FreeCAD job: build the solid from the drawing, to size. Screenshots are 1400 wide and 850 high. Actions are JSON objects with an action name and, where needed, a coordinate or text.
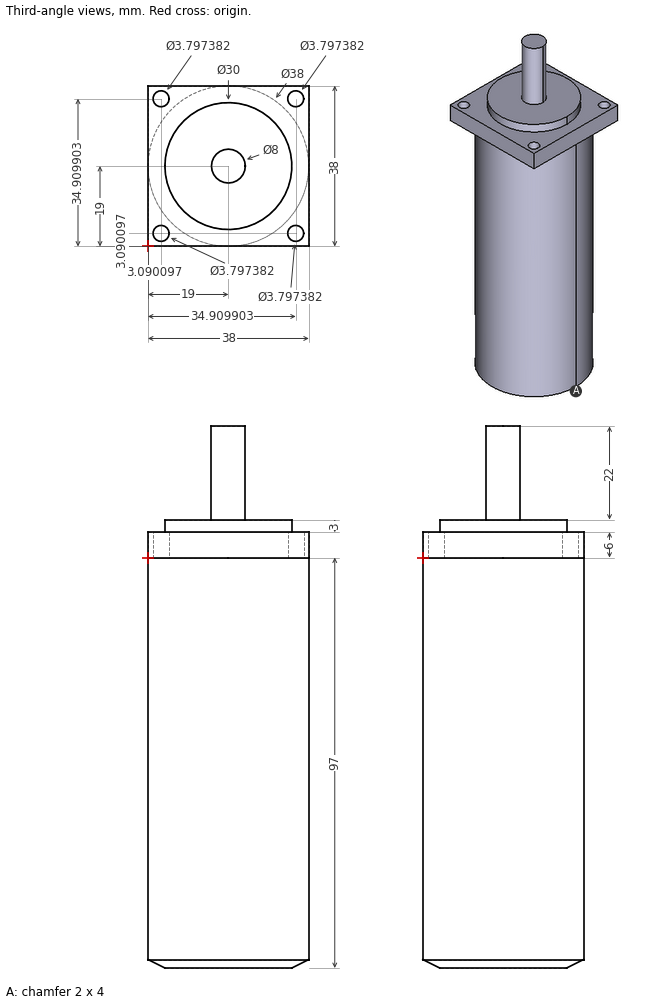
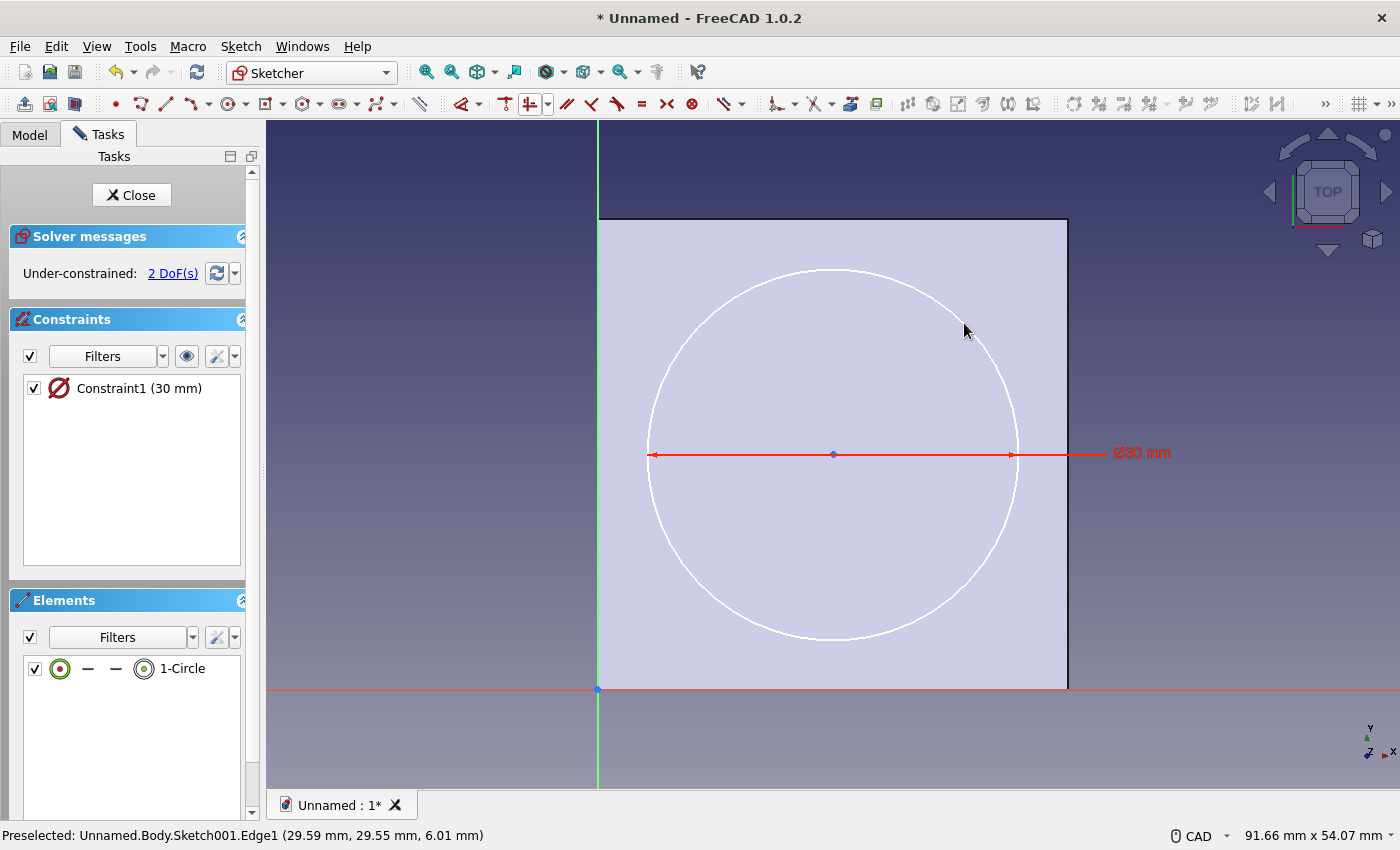
{"action": "key", "text": "d"}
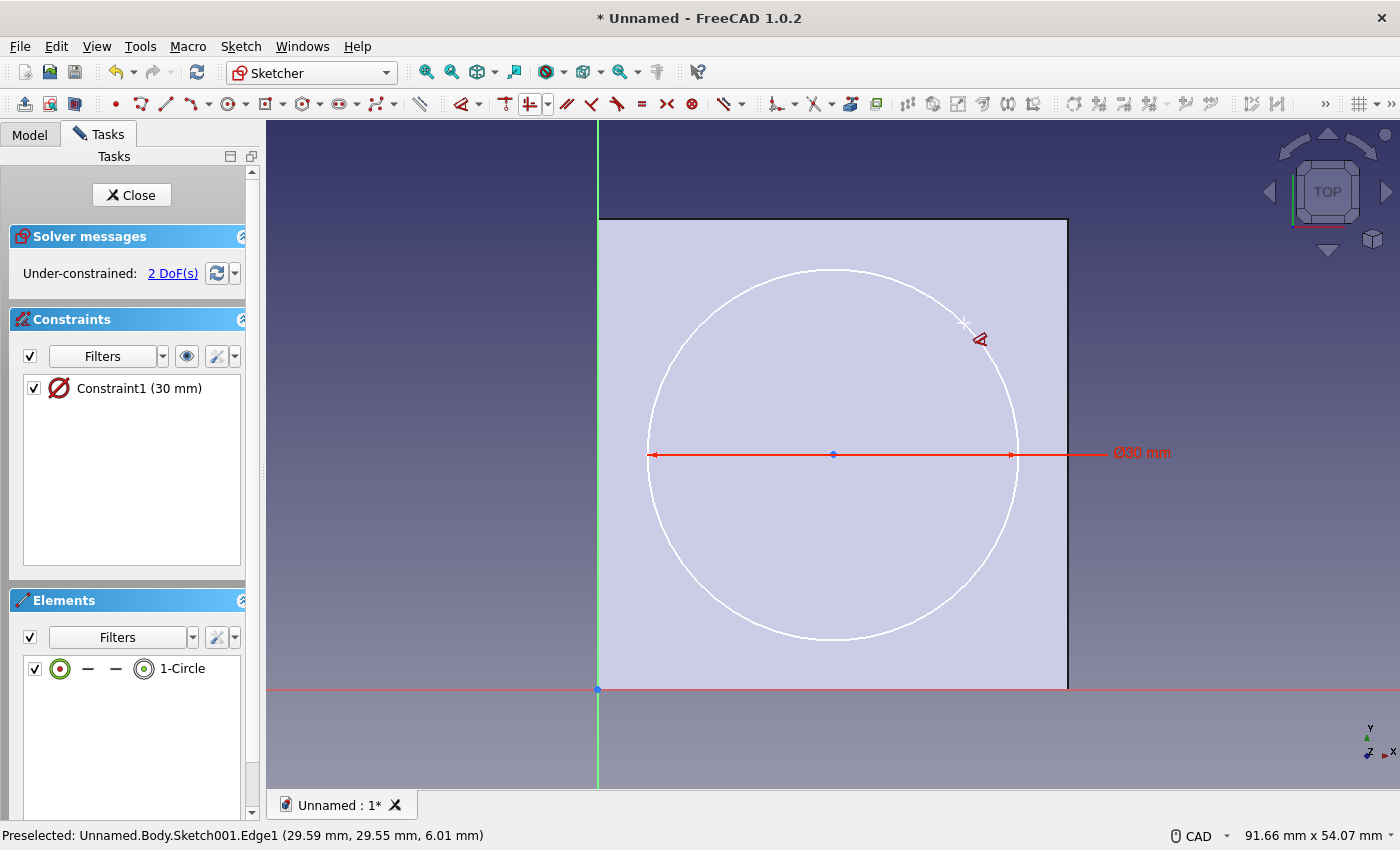
{"action": "left_click", "coordinate": [833, 455]}
{"action": "left_click", "coordinate": [715, 724]}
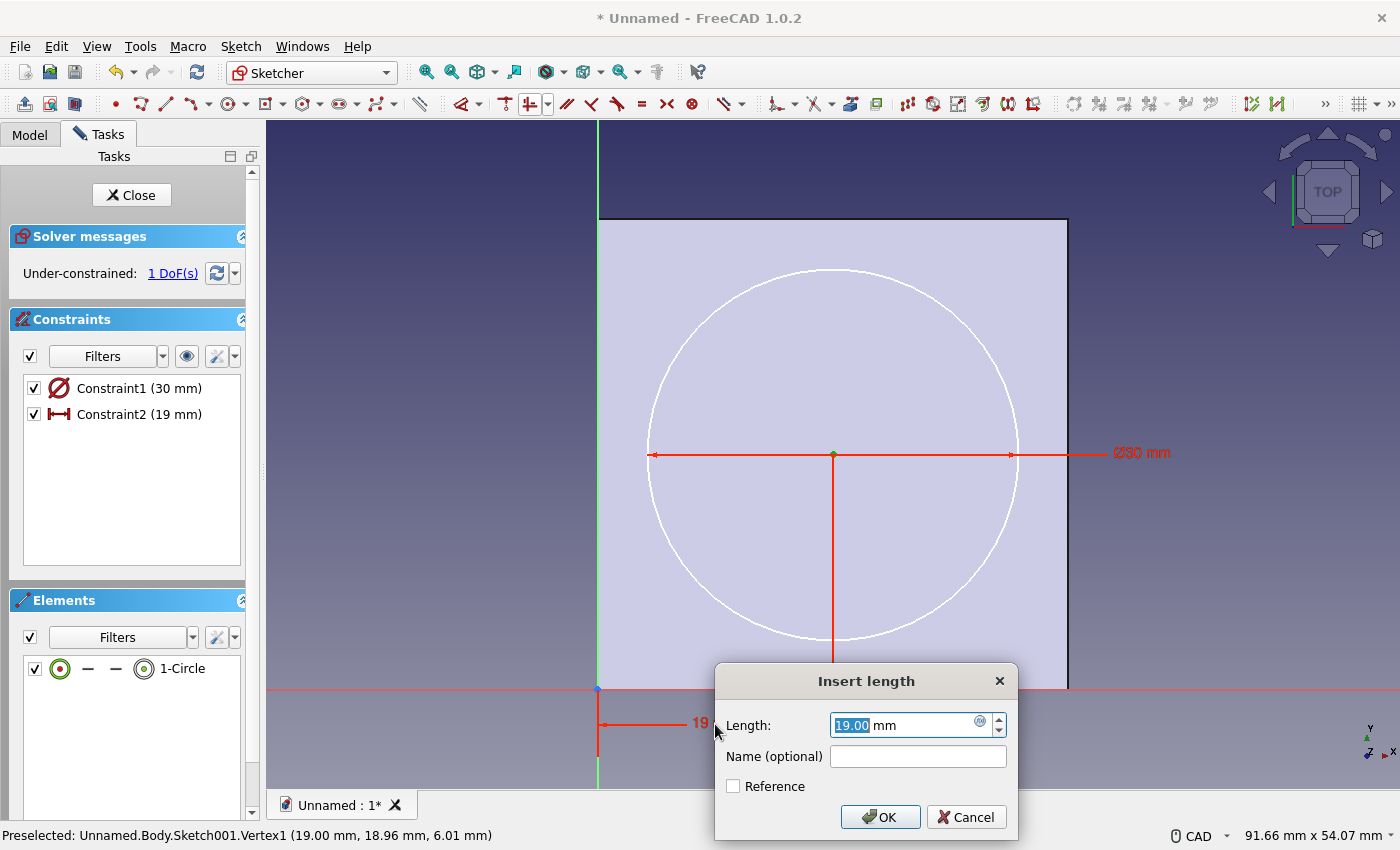
{"action": "type", "text": "19"}
{"action": "key", "text": "Return"}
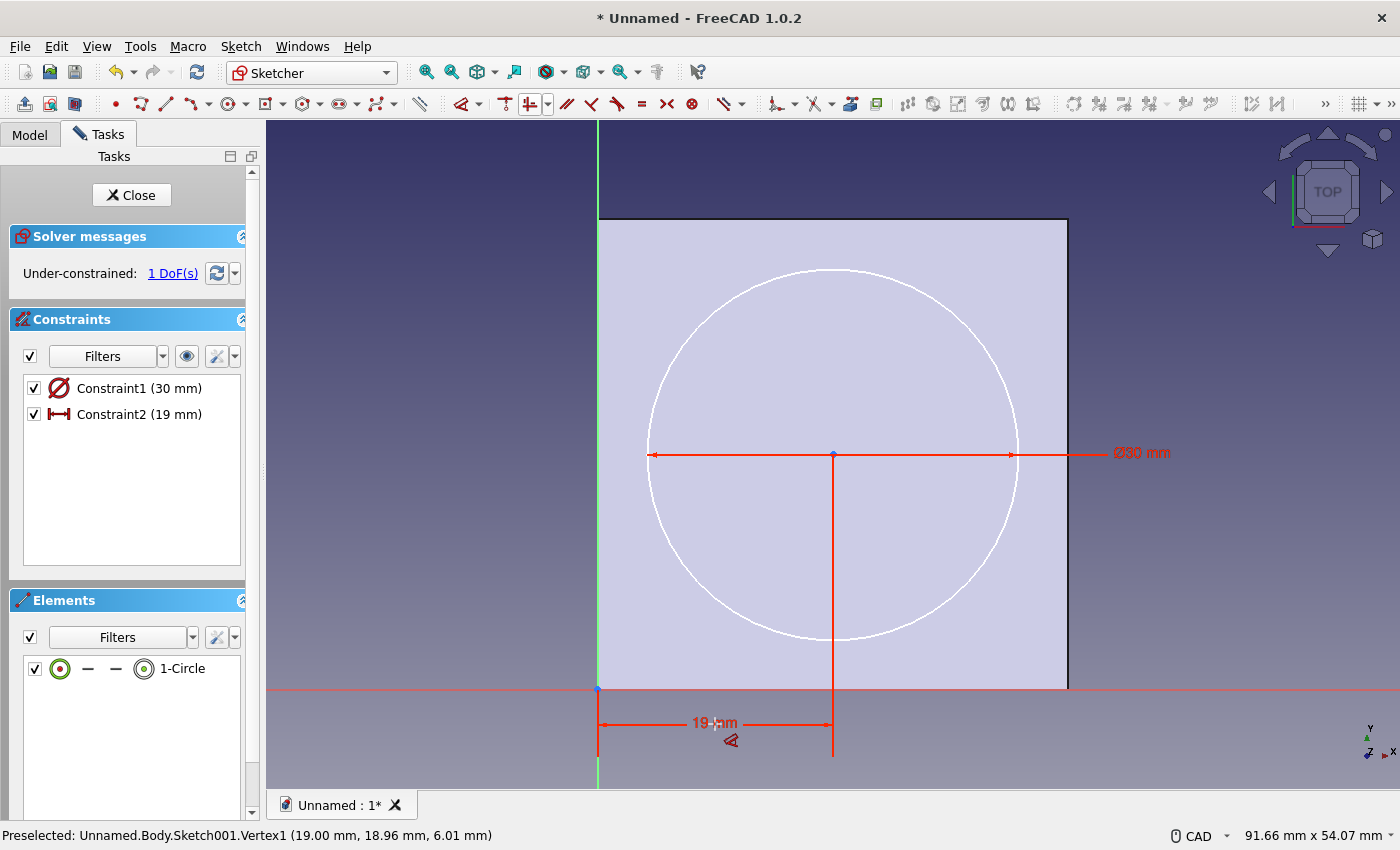
{"action": "left_click", "coordinate": [833, 455]}
{"action": "left_click", "coordinate": [564, 572]}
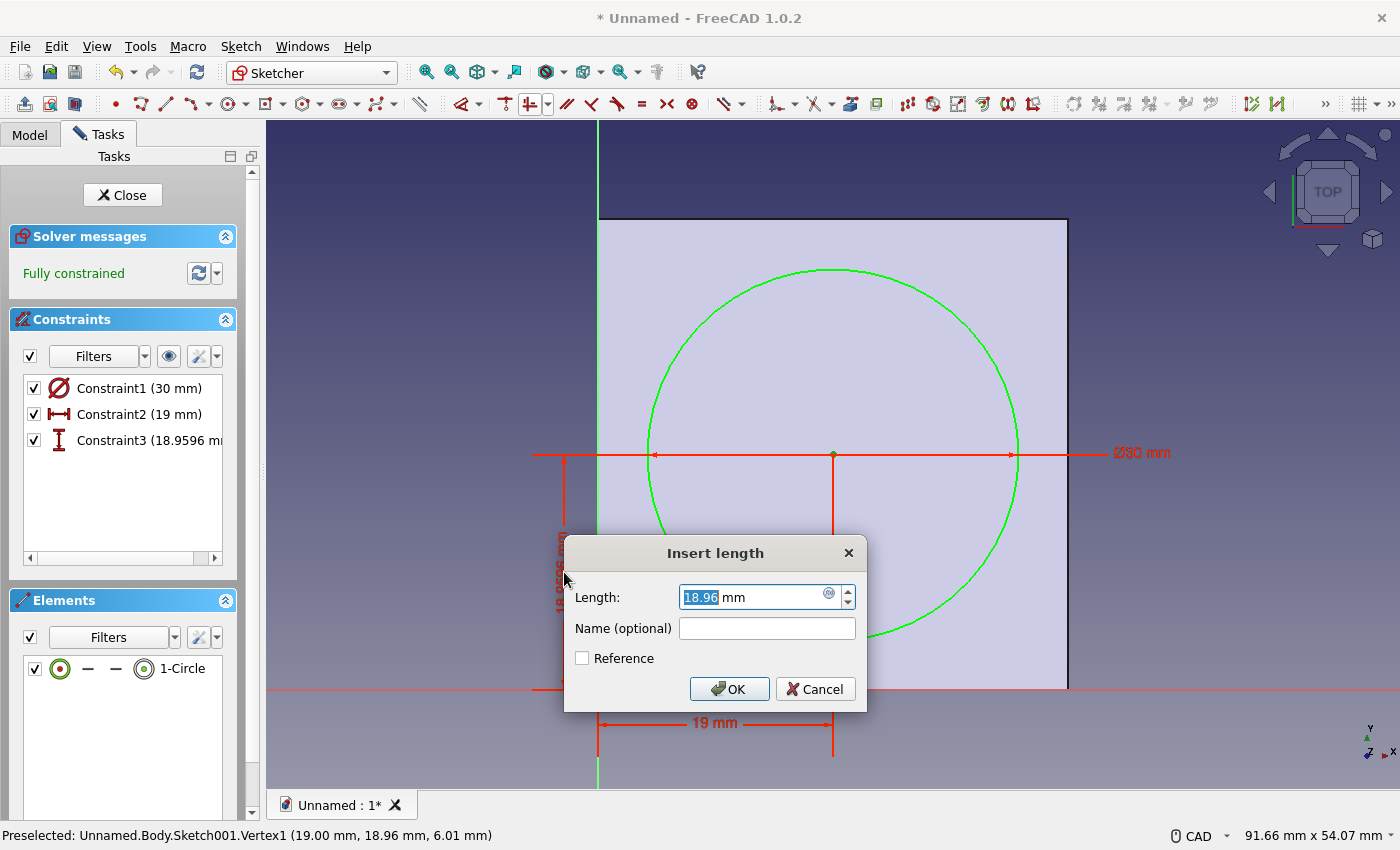
{"action": "type", "text": "19"}
{"action": "key", "text": "Return"}
{"action": "key", "text": "Escape"}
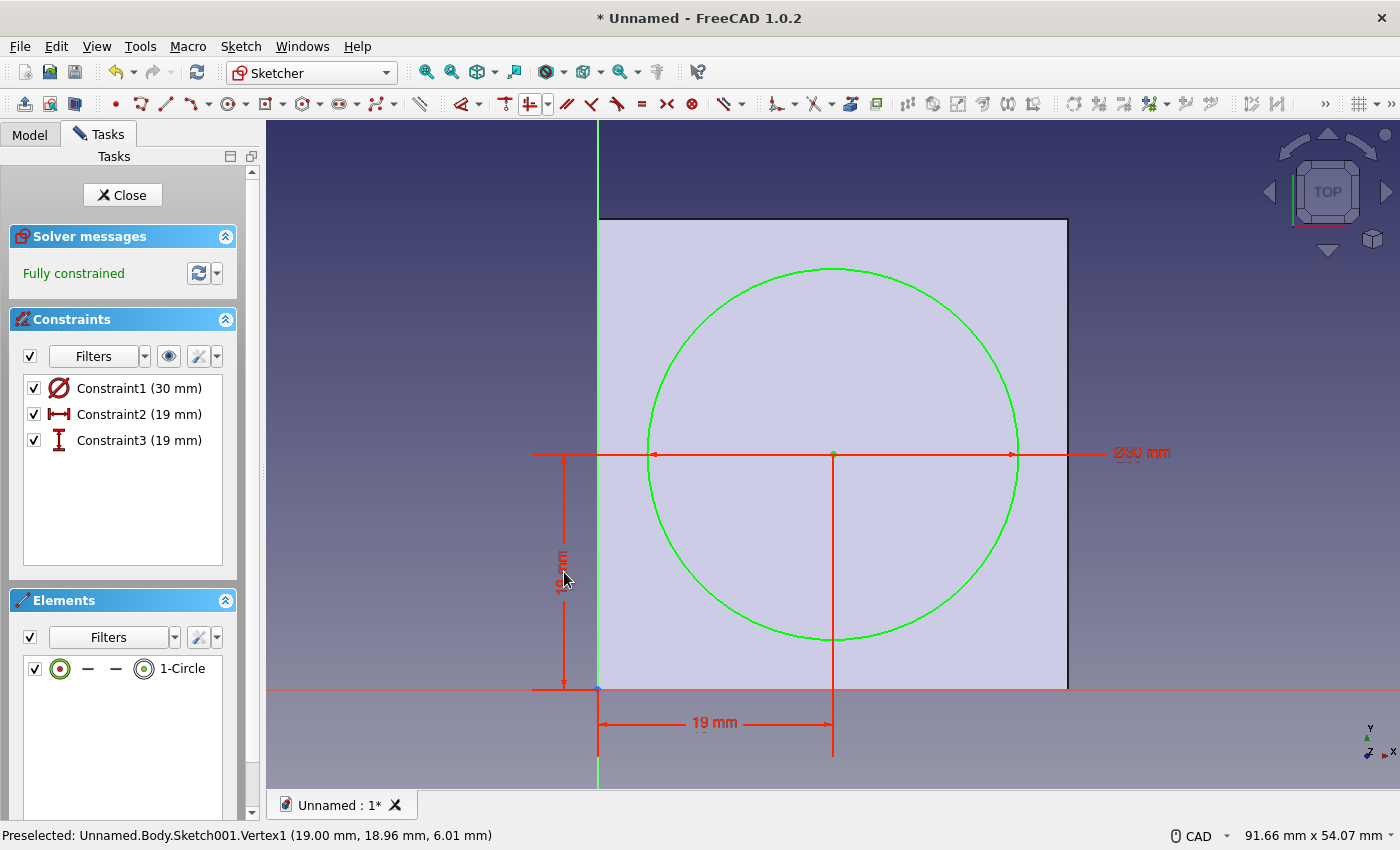
{"action": "left_click", "coordinate": [123, 195]}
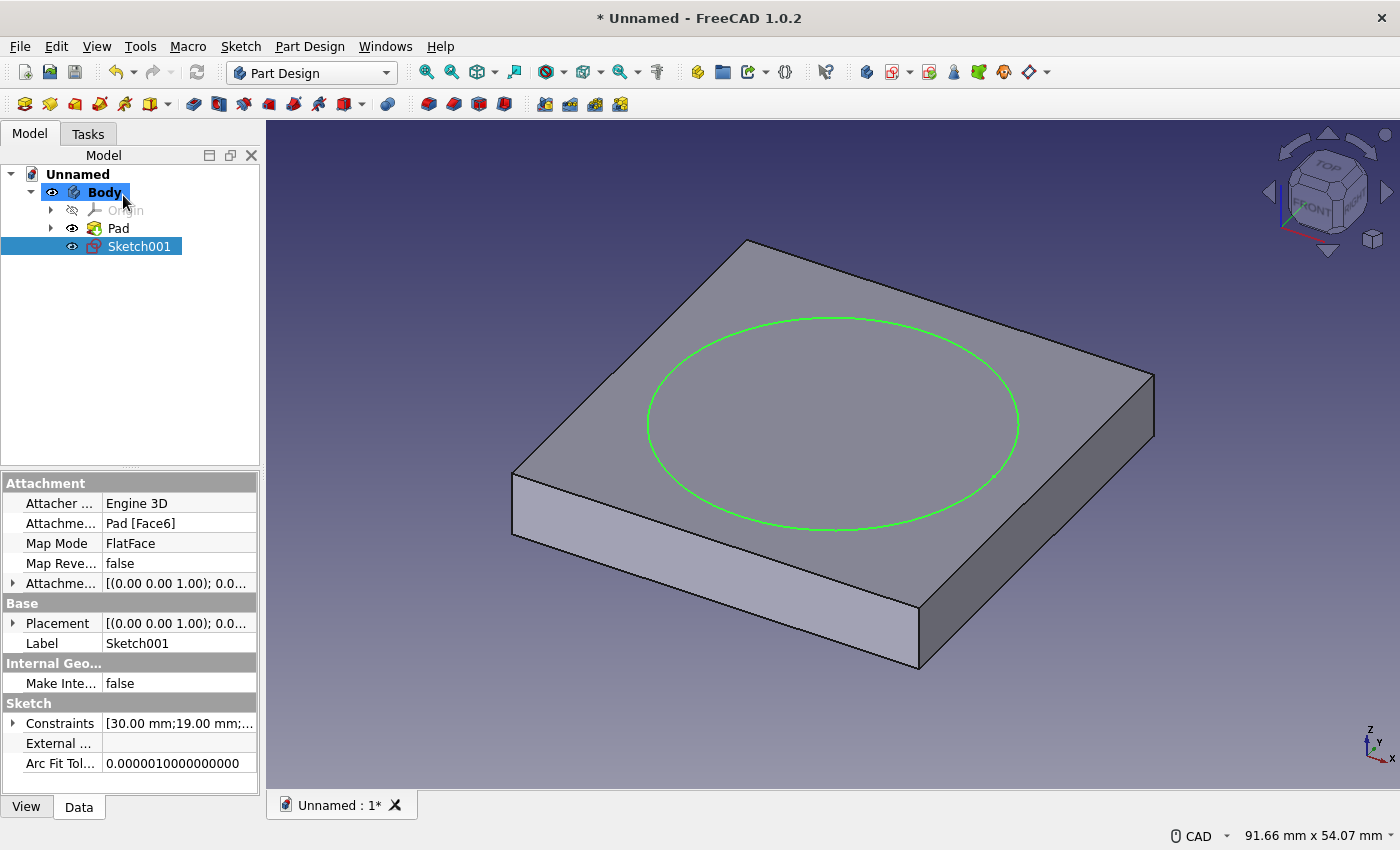
{"action": "left_click", "coordinate": [25, 104]}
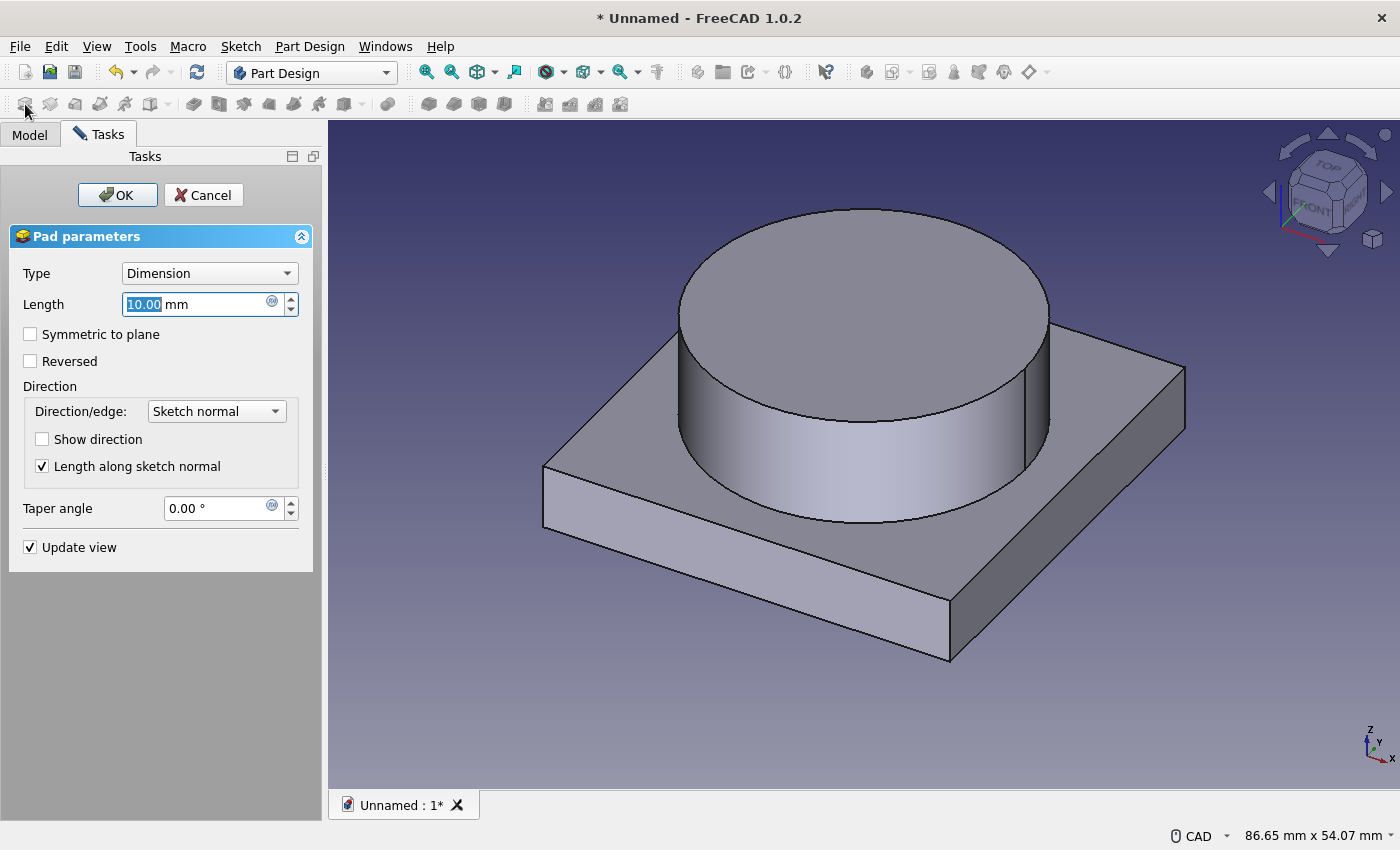
{"action": "type", "text": "3"}
{"action": "key", "text": "Tab"}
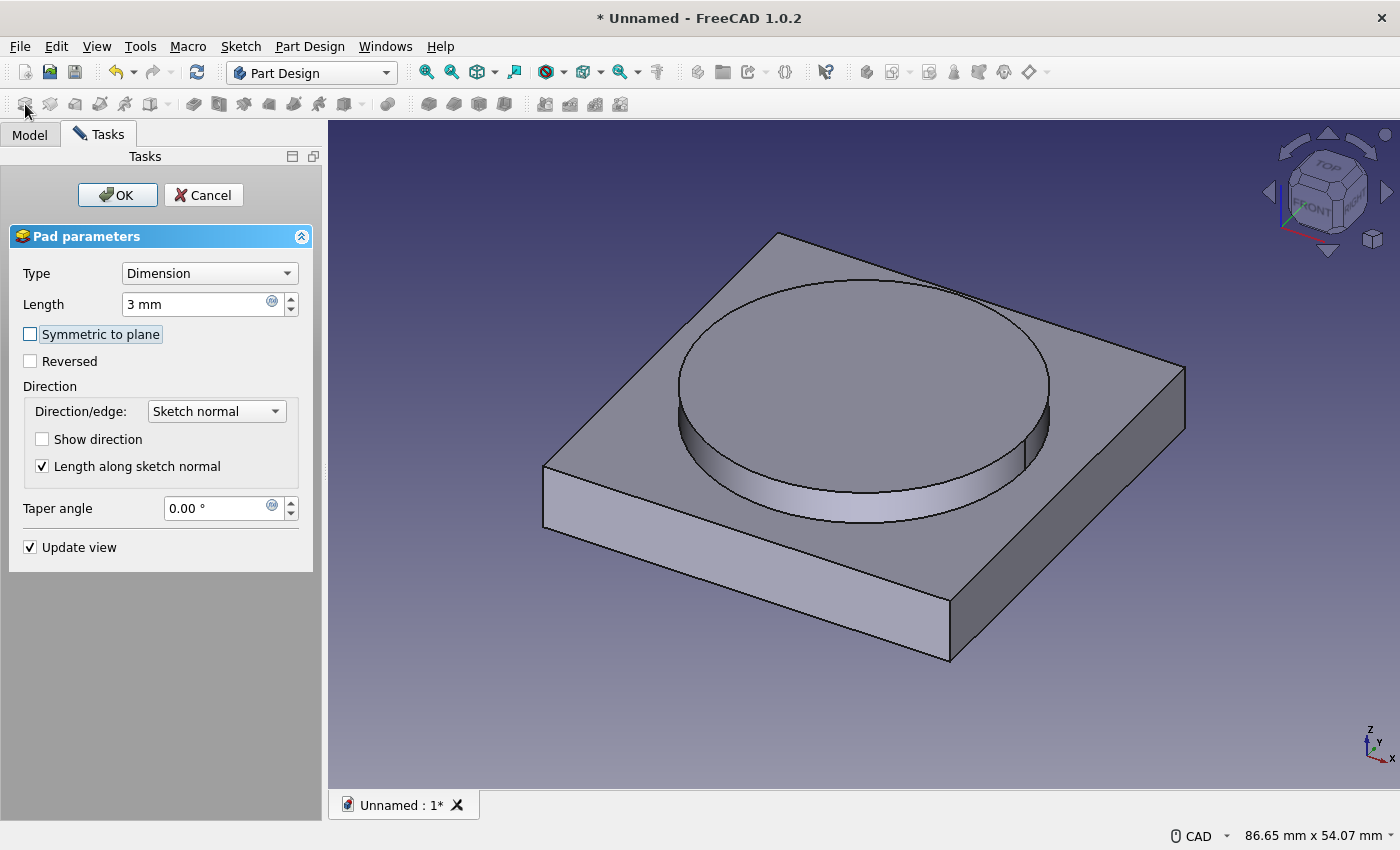
{"action": "left_click", "coordinate": [118, 195]}